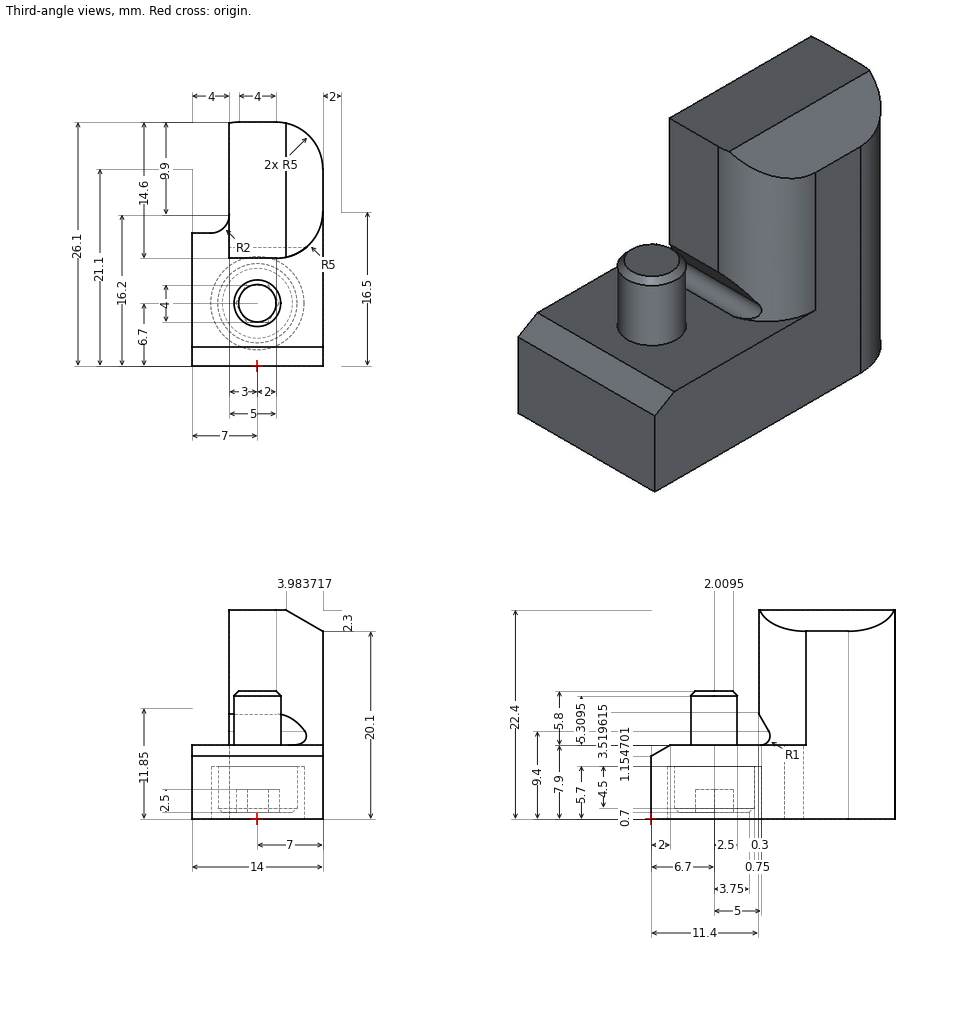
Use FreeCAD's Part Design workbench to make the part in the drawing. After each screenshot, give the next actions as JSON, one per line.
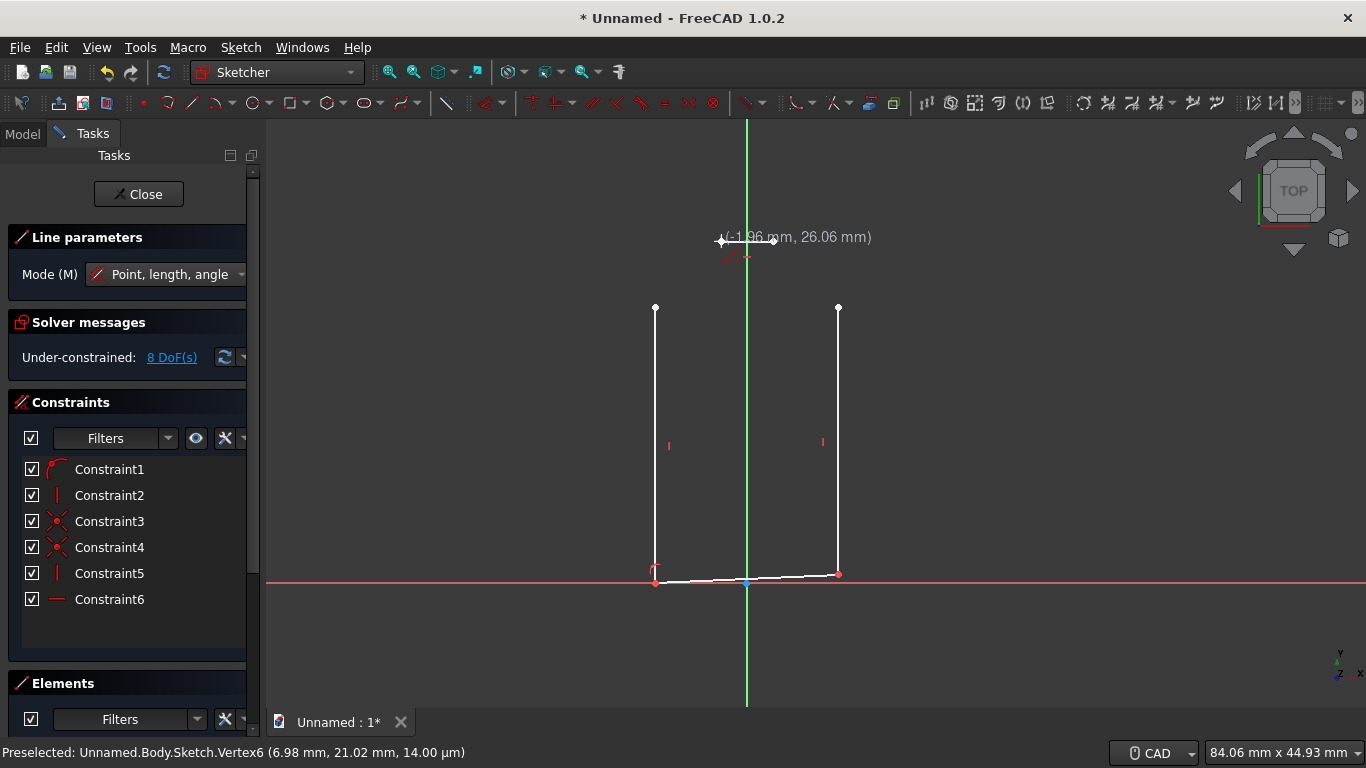
{"action": "key", "text": "g 3 a"}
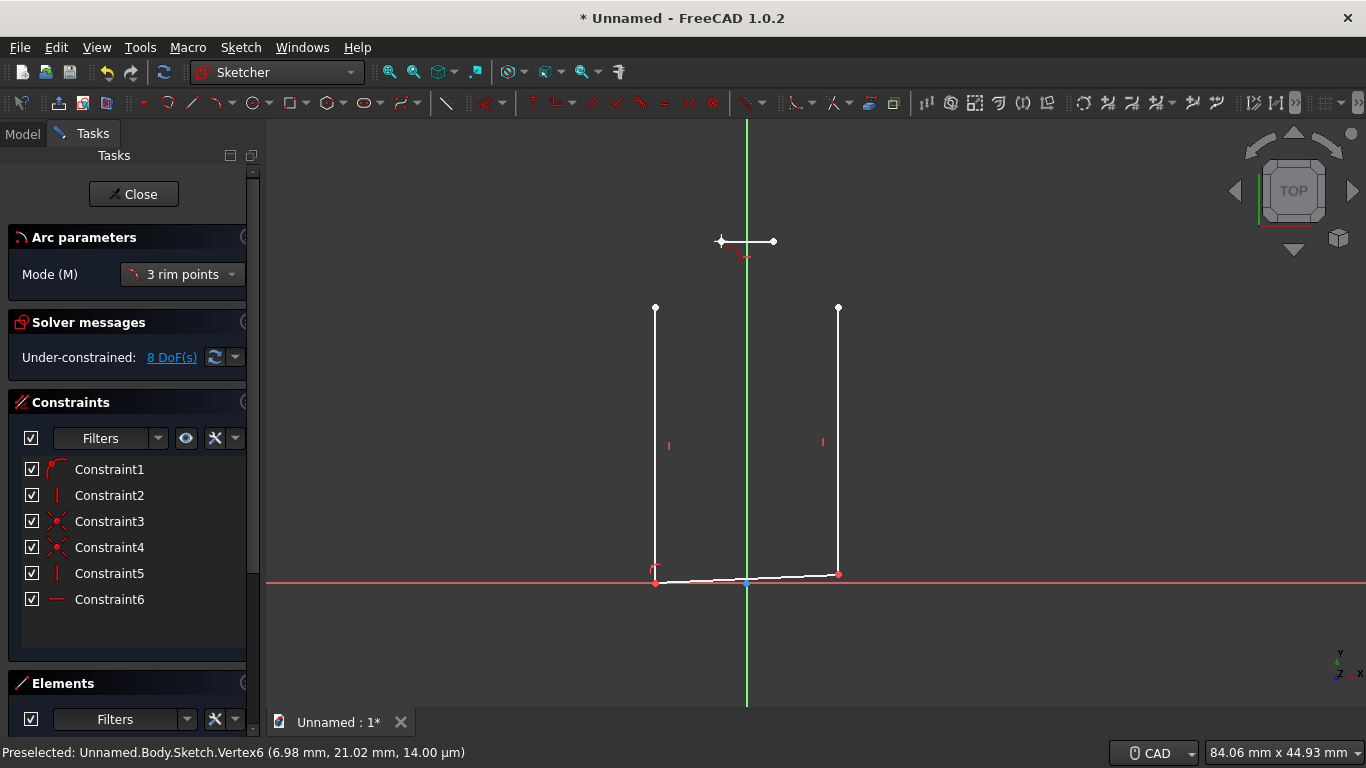
{"action": "left_click", "coordinate": [838, 308]}
{"action": "left_click", "coordinate": [773, 242]}
{"action": "left_click", "coordinate": [819, 261]}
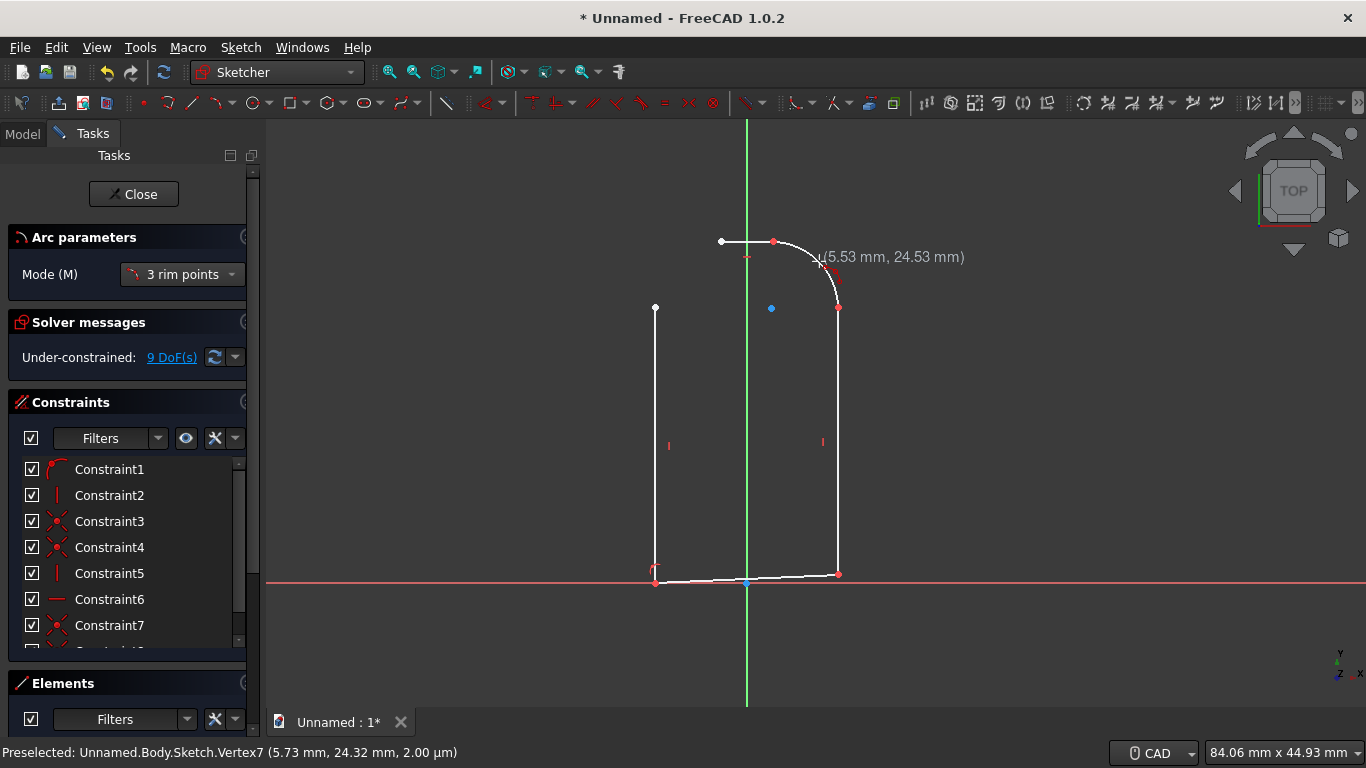
{"action": "left_click", "coordinate": [721, 242]}
{"action": "left_click", "coordinate": [655, 308]}
{"action": "left_click", "coordinate": [674, 261]}
{"action": "key", "text": "Escape"}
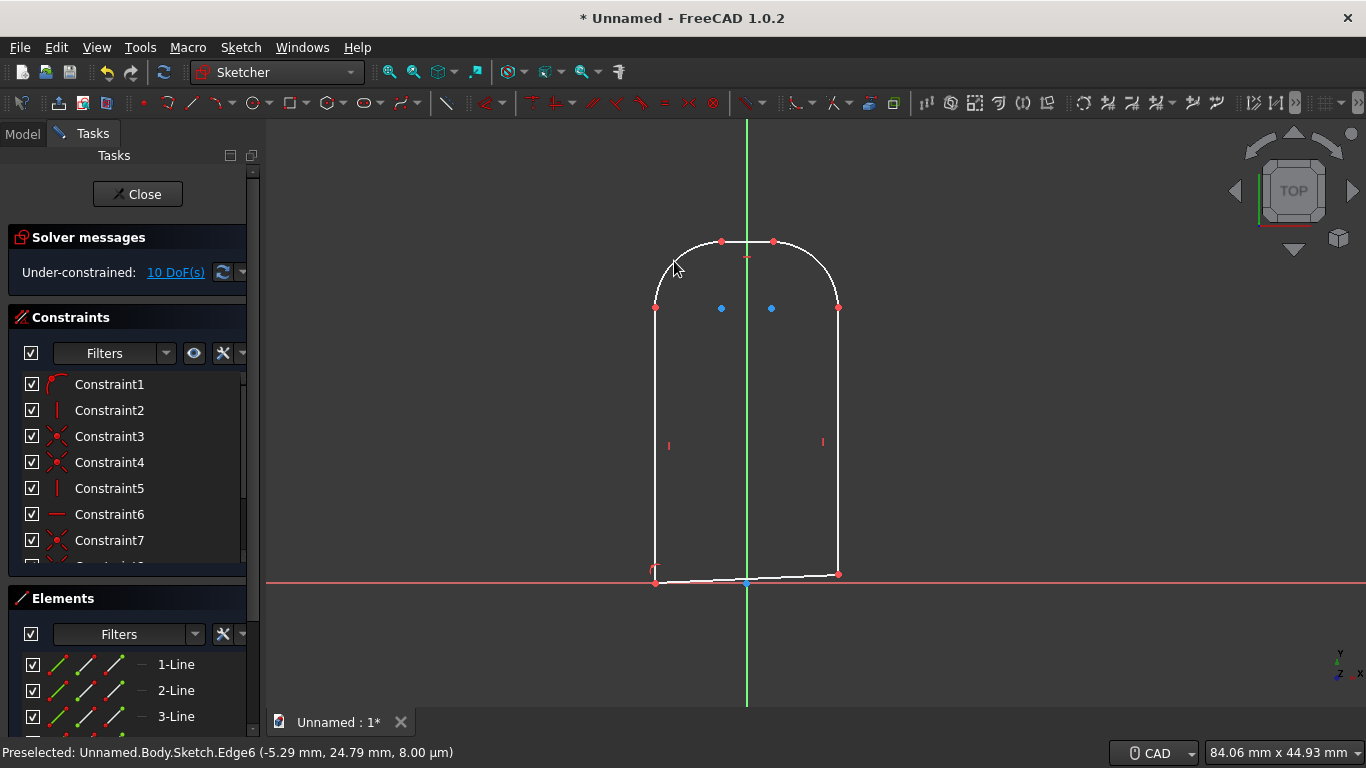
{"action": "left_click", "coordinate": [655, 391]}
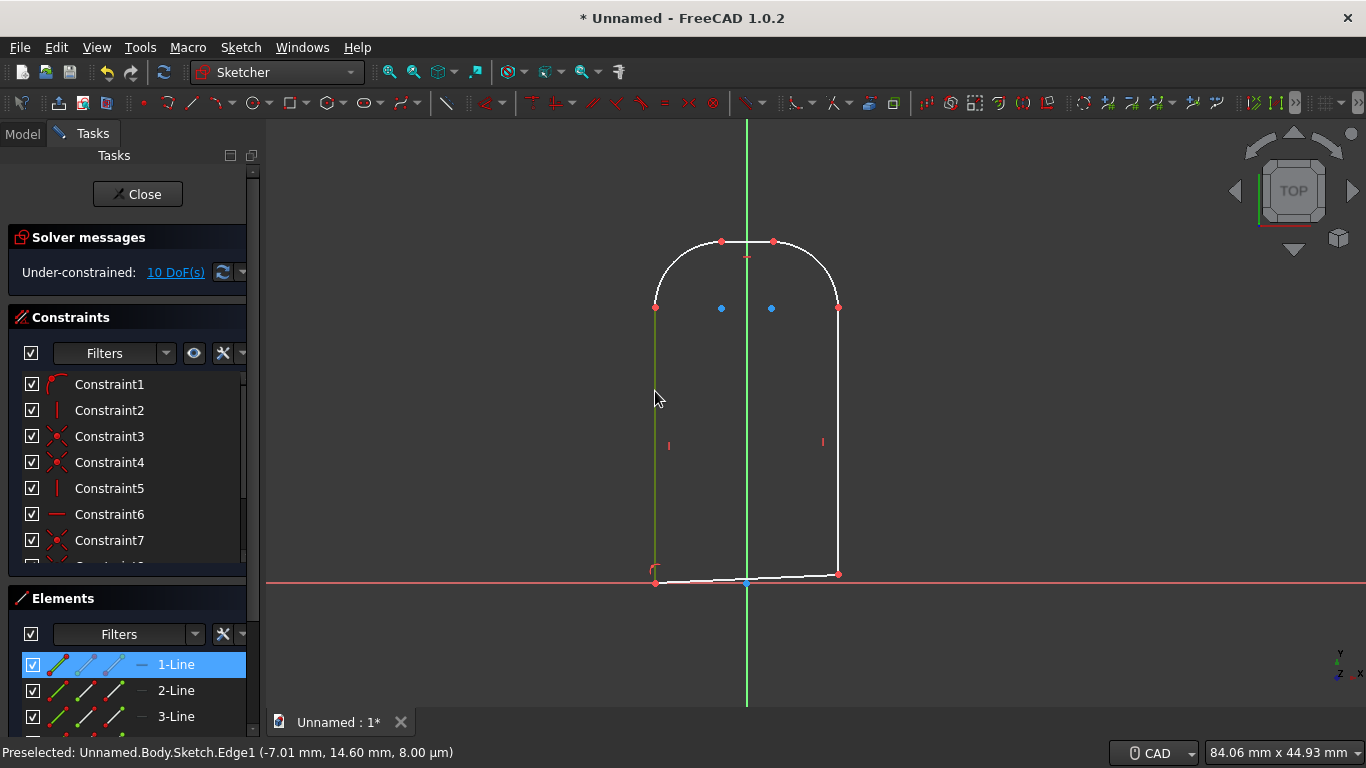
{"action": "left_click", "coordinate": [691, 249]}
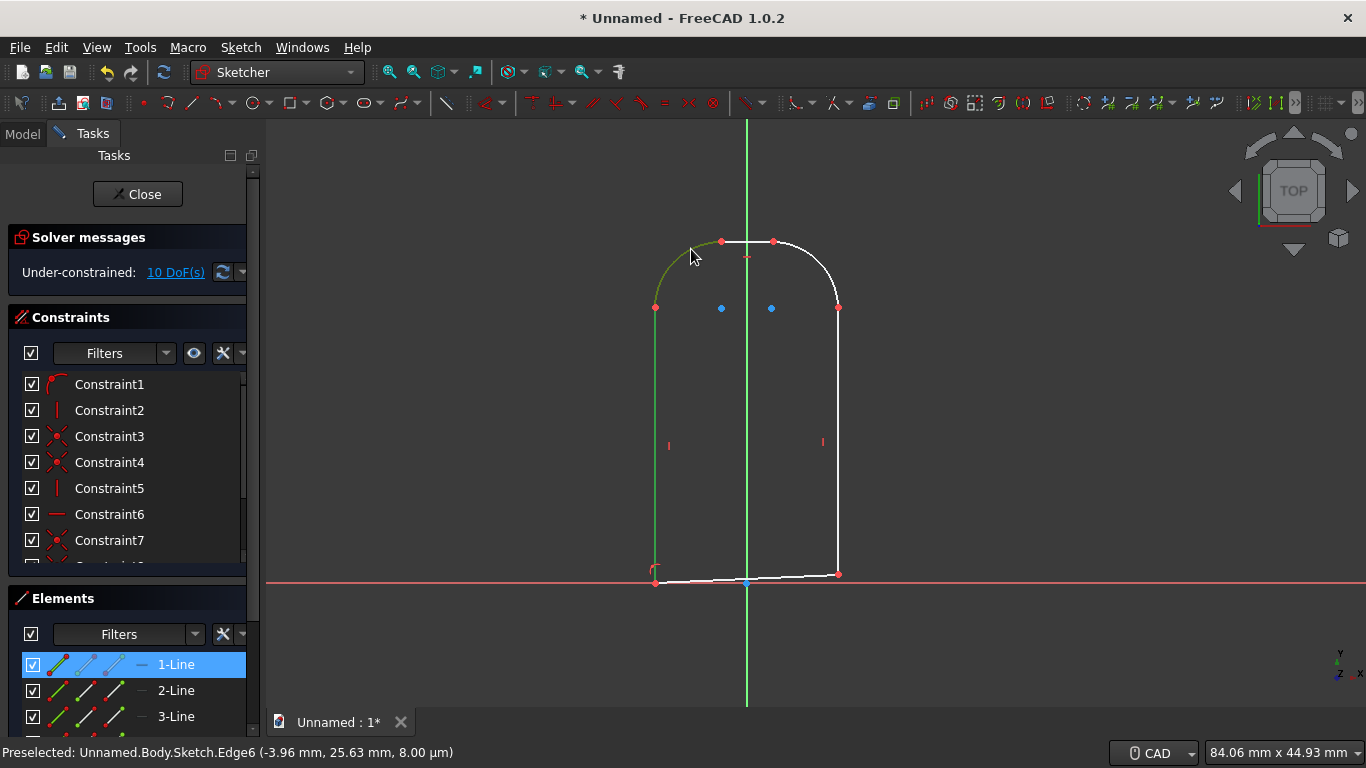
{"action": "left_click", "coordinate": [642, 104]}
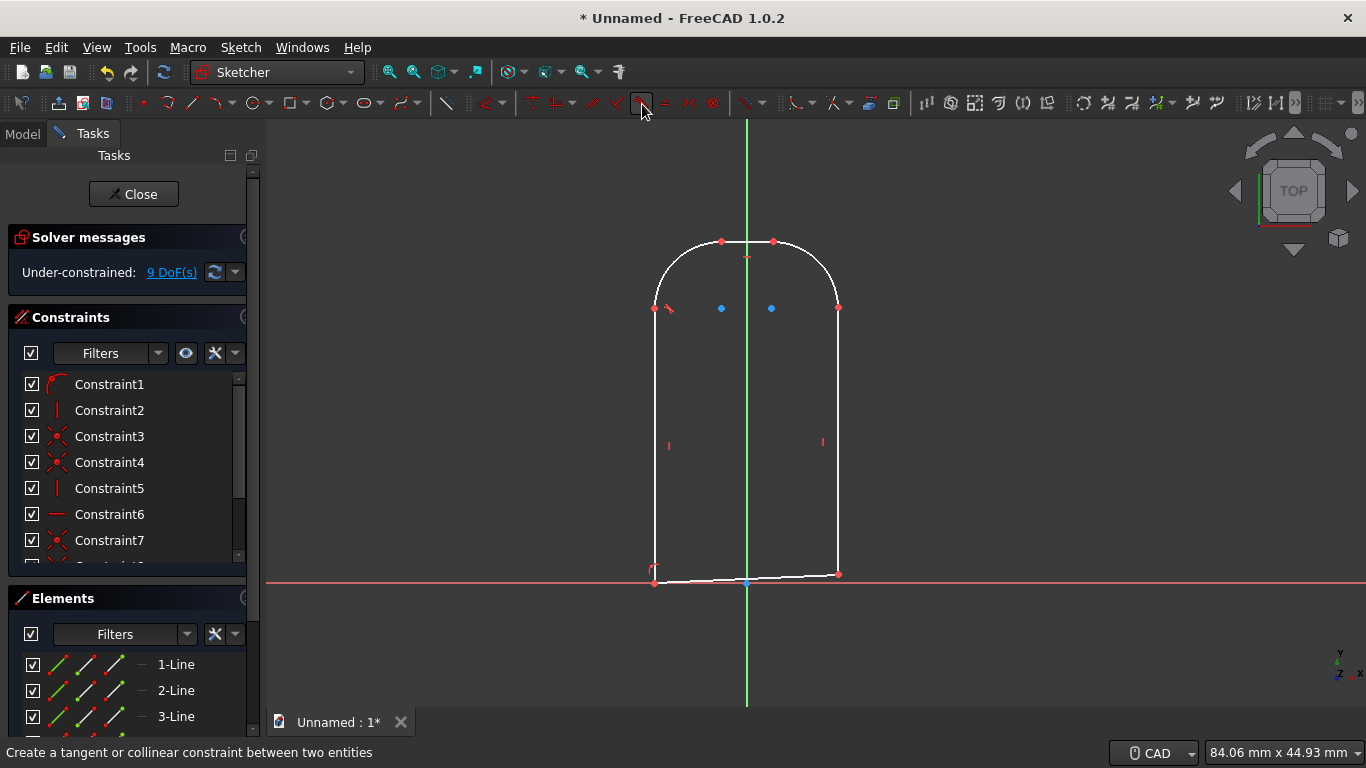
{"action": "left_click", "coordinate": [838, 495]}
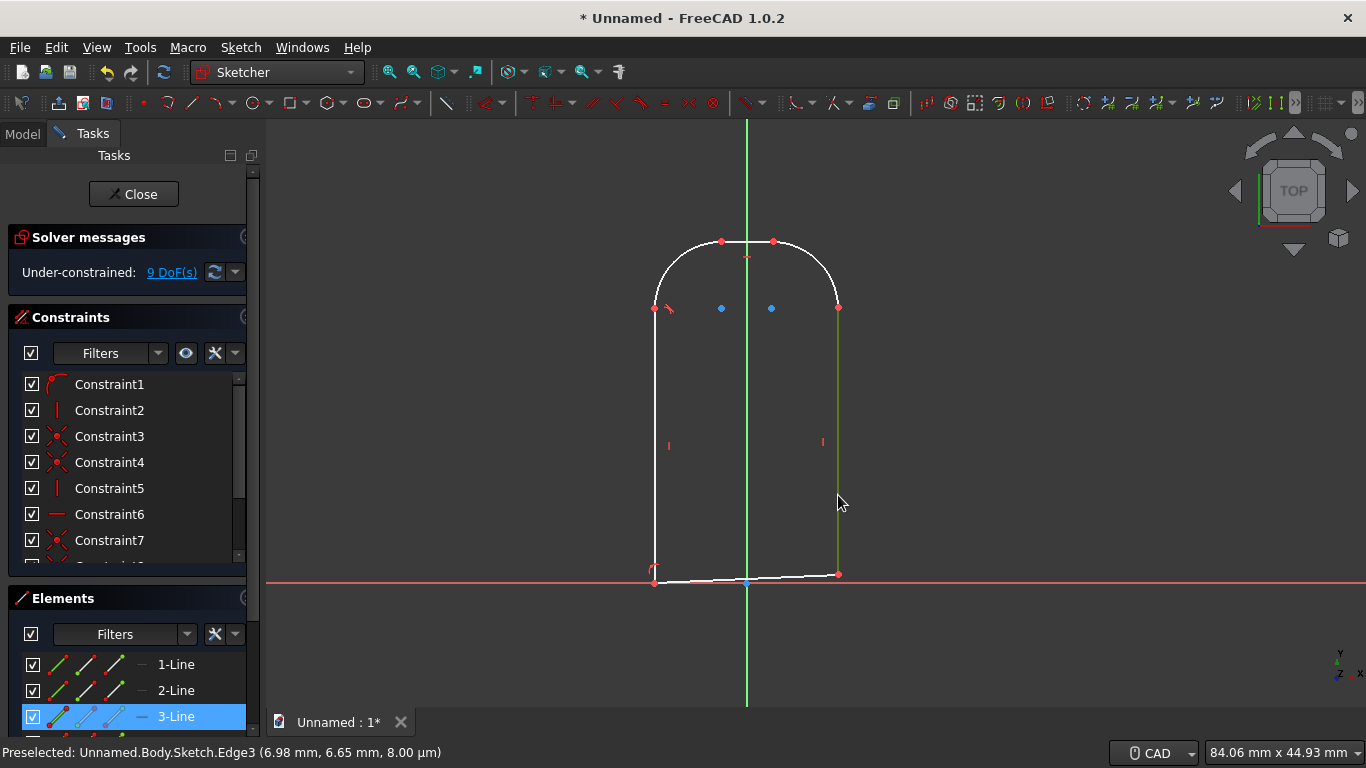
{"action": "left_click", "coordinate": [831, 278]}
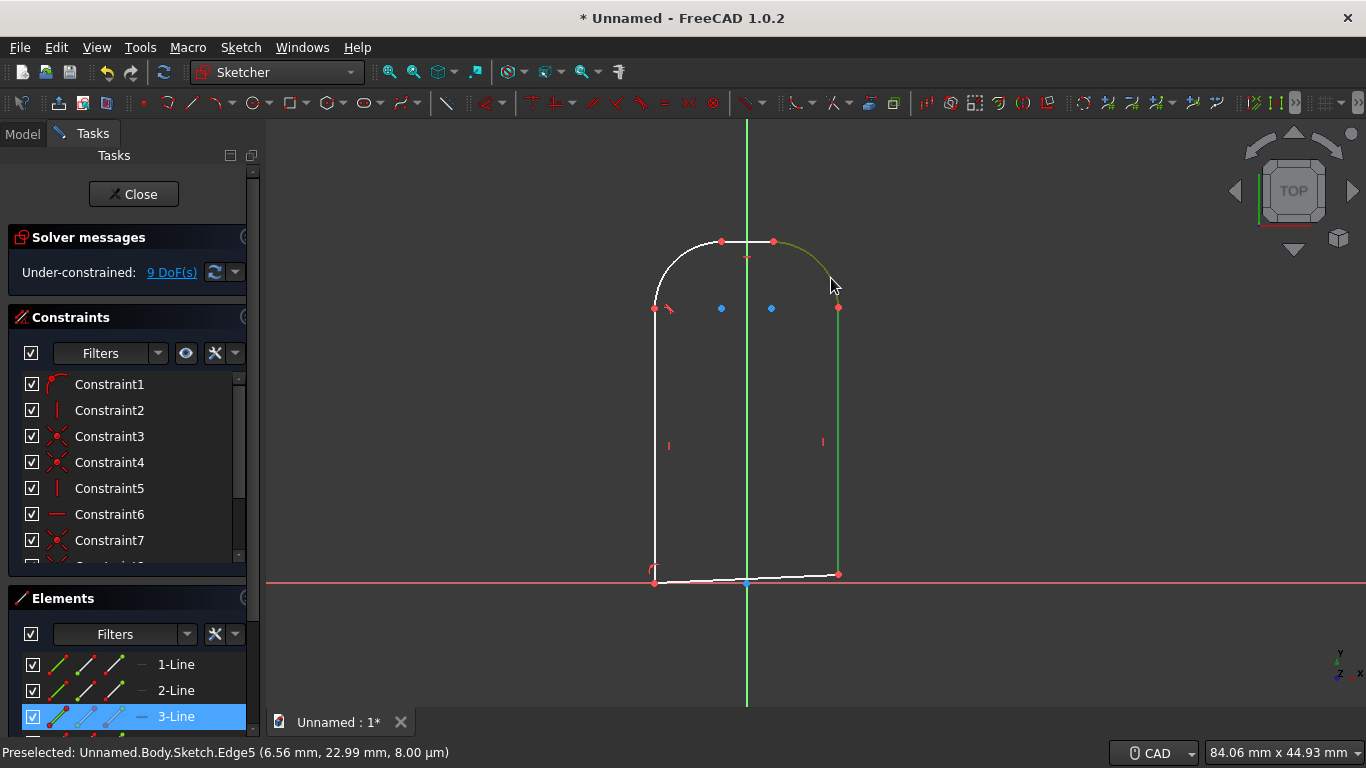
{"action": "left_click", "coordinate": [642, 104]}